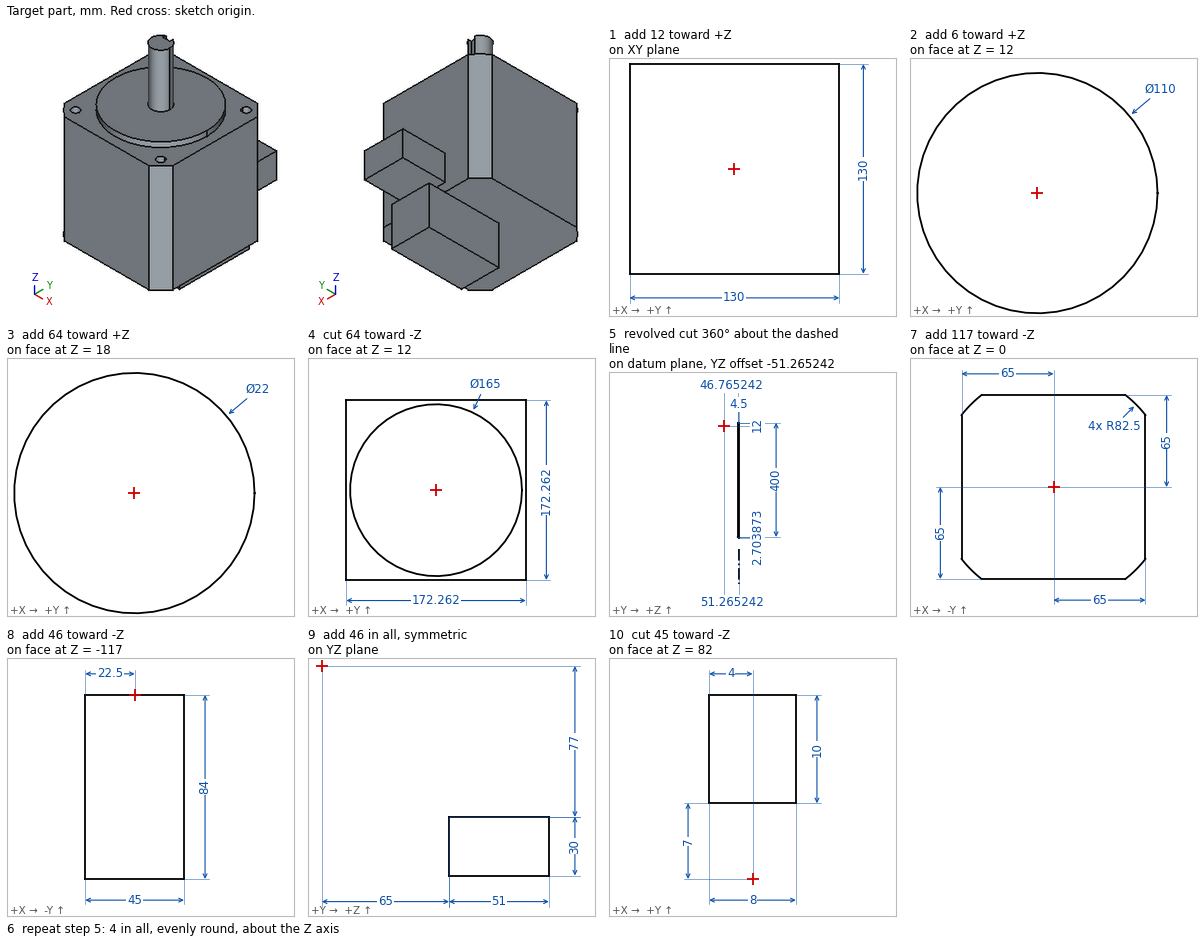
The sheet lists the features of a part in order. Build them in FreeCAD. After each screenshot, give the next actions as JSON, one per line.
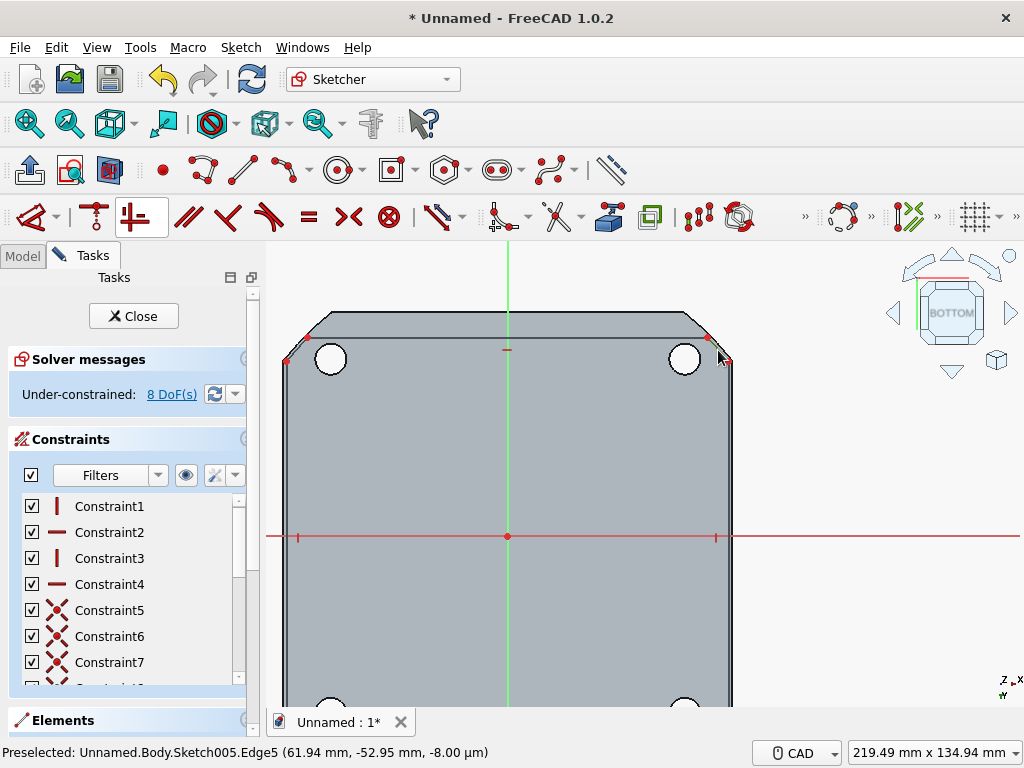
{"action": "scroll", "coordinate": [301, 345], "scroll_direction": "up", "scroll_amount": 2}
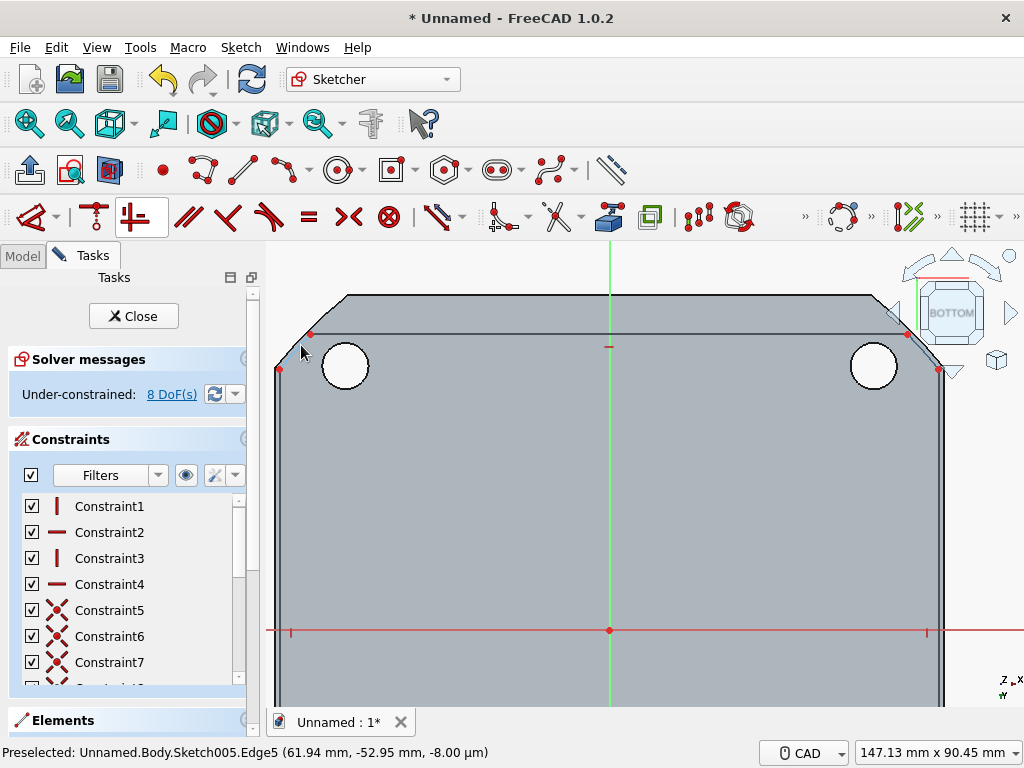
{"action": "left_click", "coordinate": [301, 345]}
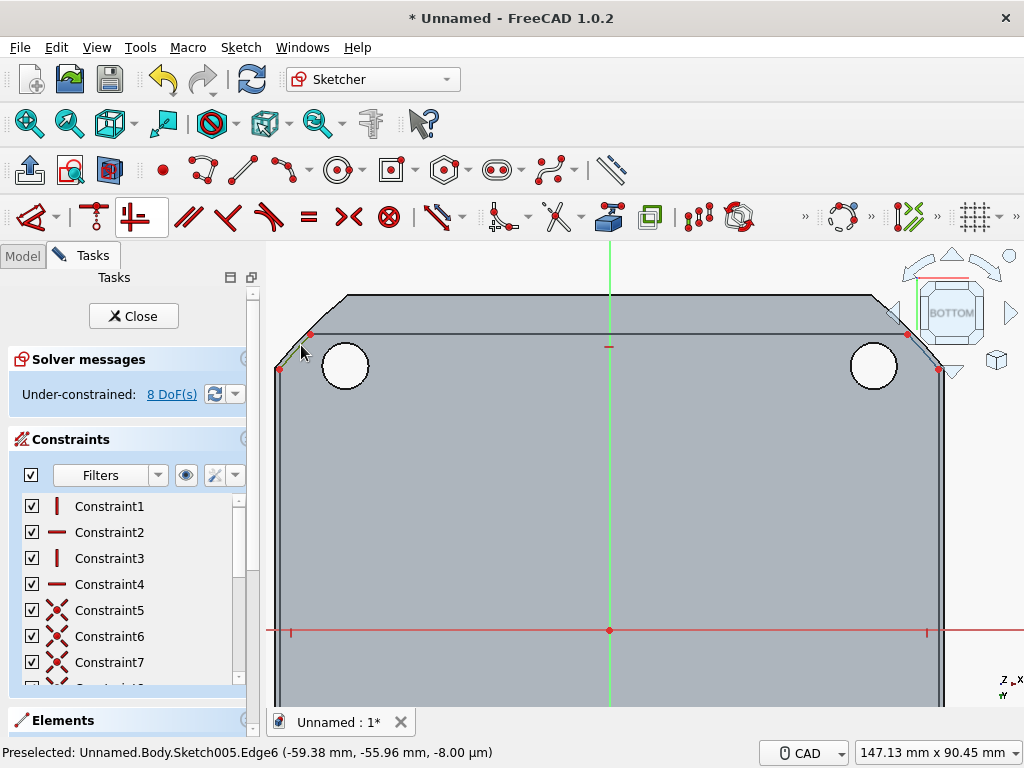
{"action": "scroll", "coordinate": [550, 347], "scroll_direction": "down", "scroll_amount": 4}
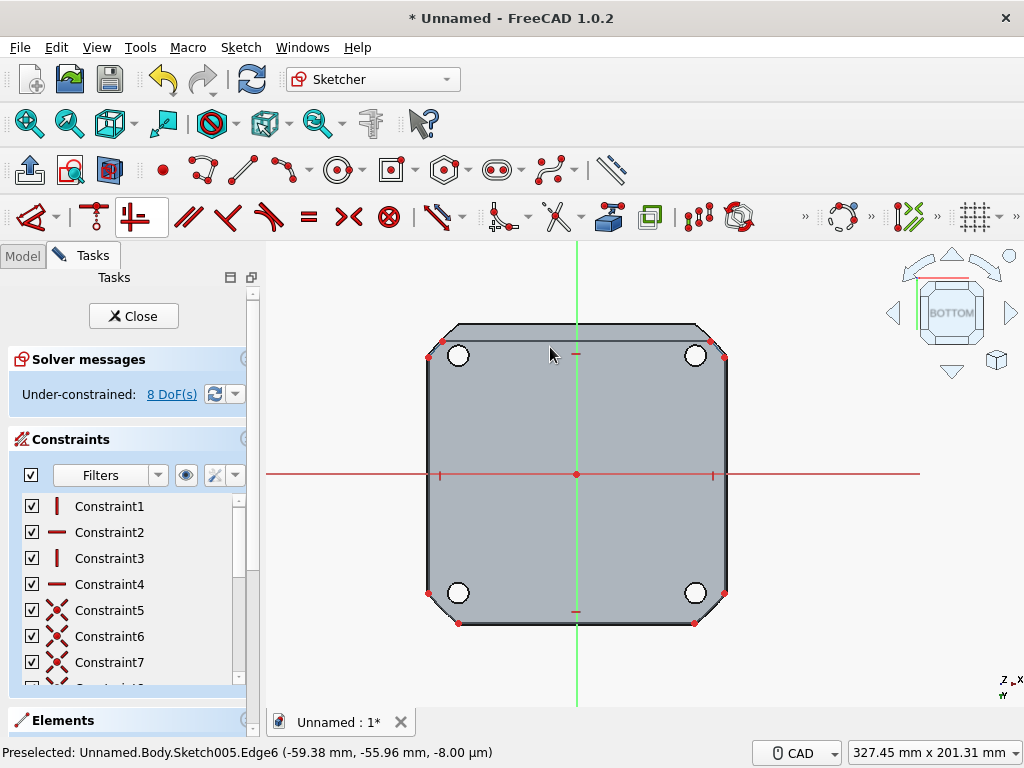
{"action": "left_click", "coordinate": [437, 603]}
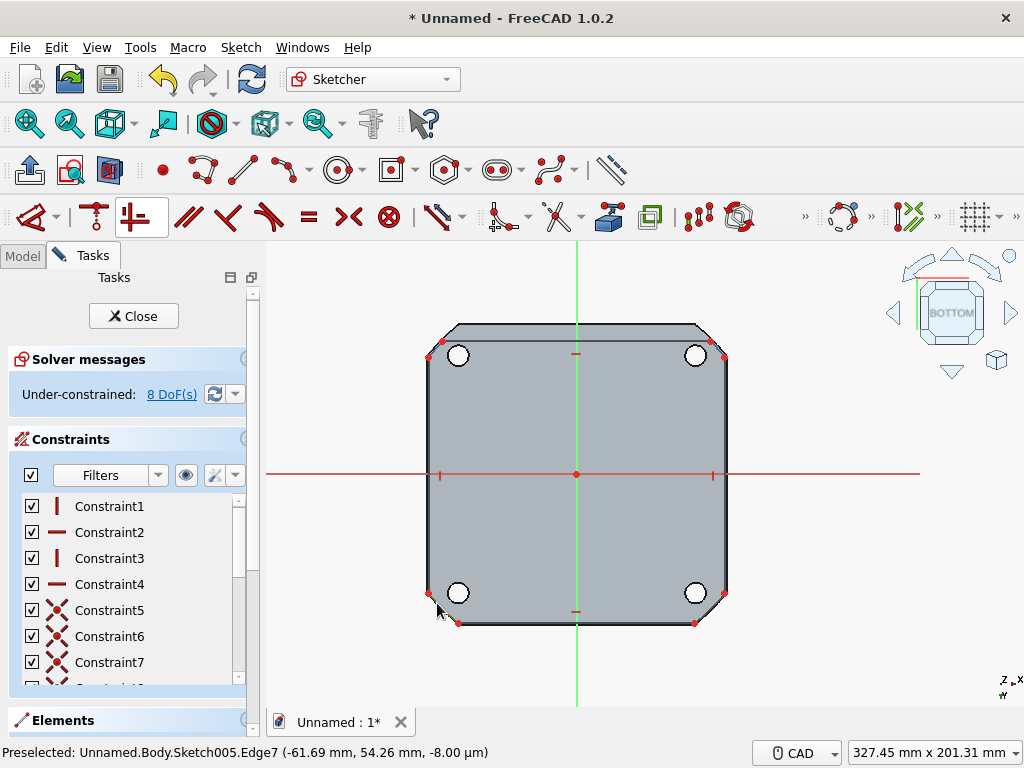
{"action": "left_click", "coordinate": [704, 615]}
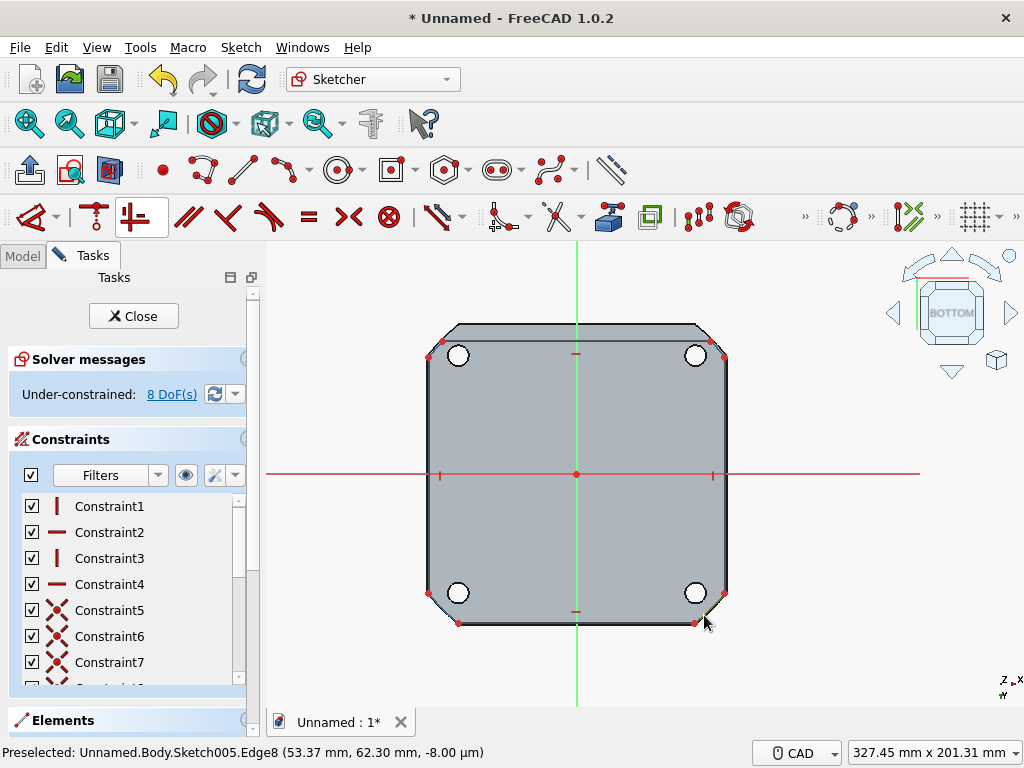
{"action": "left_click", "coordinate": [310, 218]}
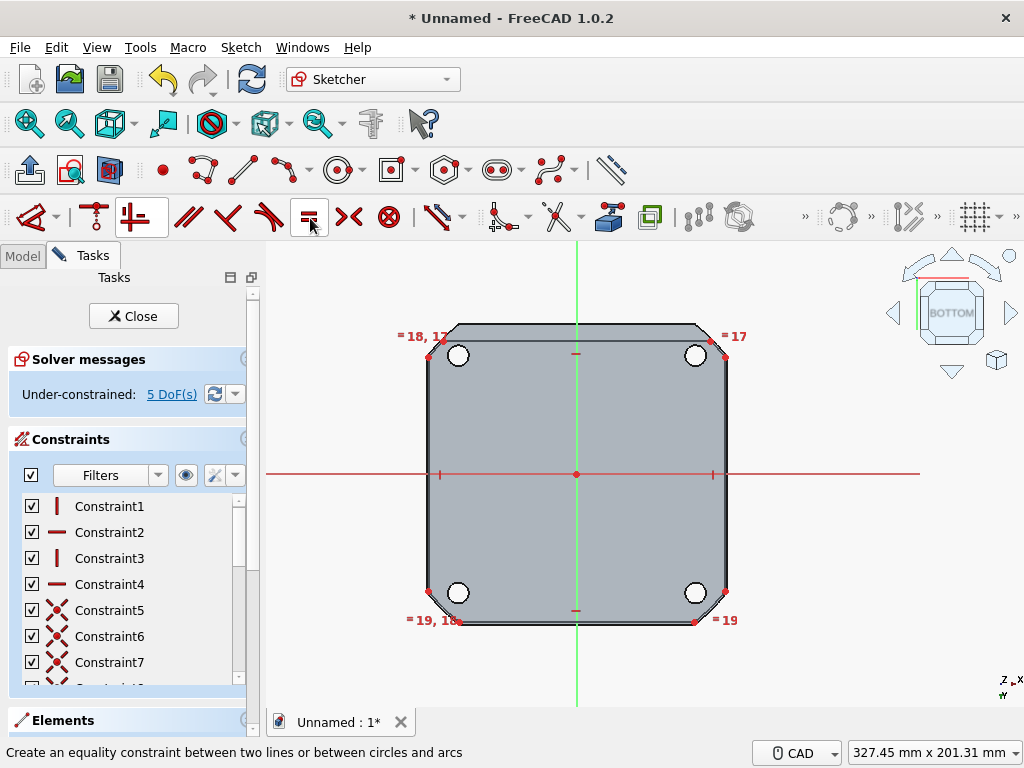
{"action": "left_click", "coordinate": [32, 218]}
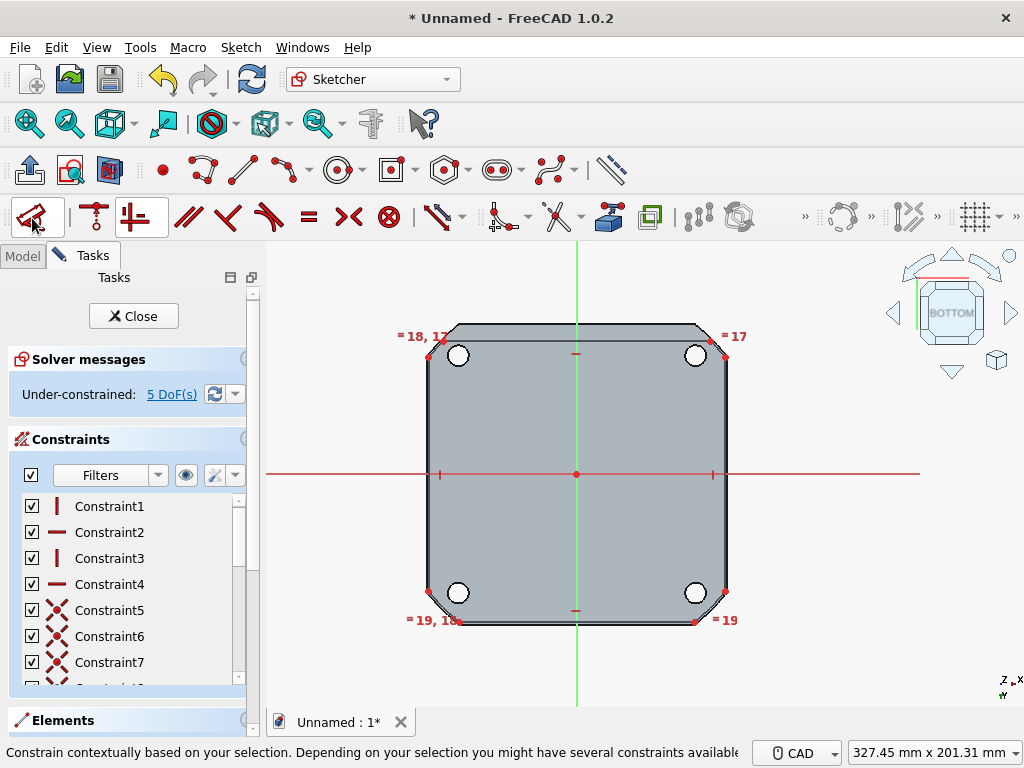
{"action": "scroll", "coordinate": [718, 349], "scroll_direction": "up", "scroll_amount": 2}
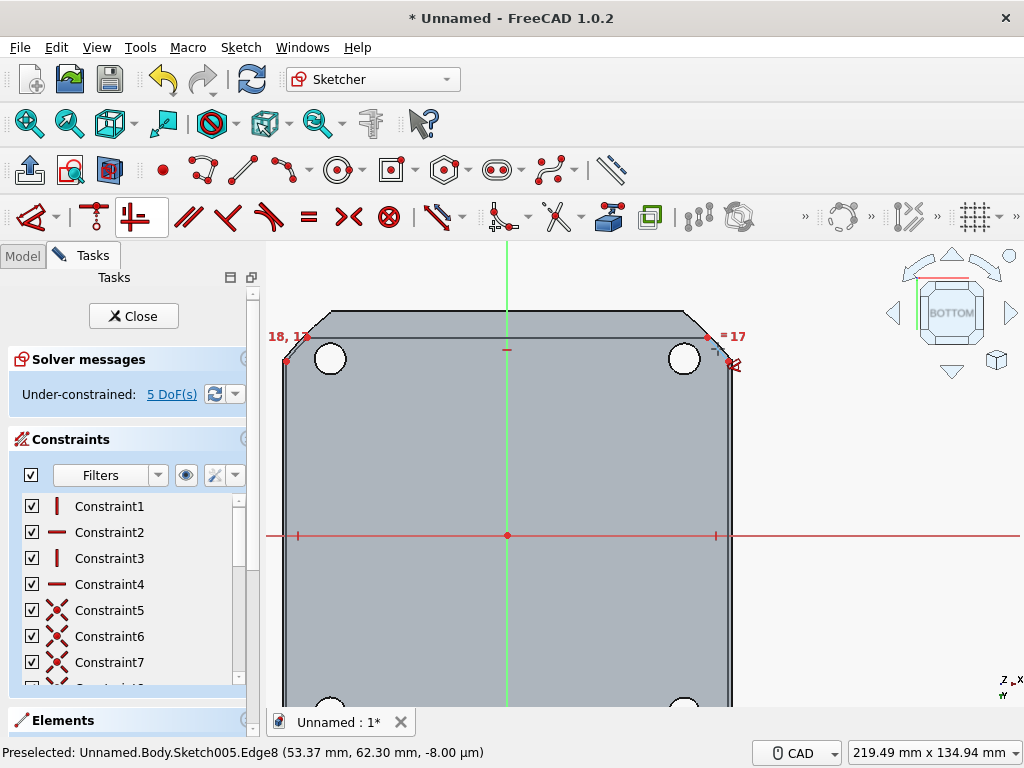
{"action": "left_click", "coordinate": [718, 349]}
{"action": "left_click", "coordinate": [742, 328]}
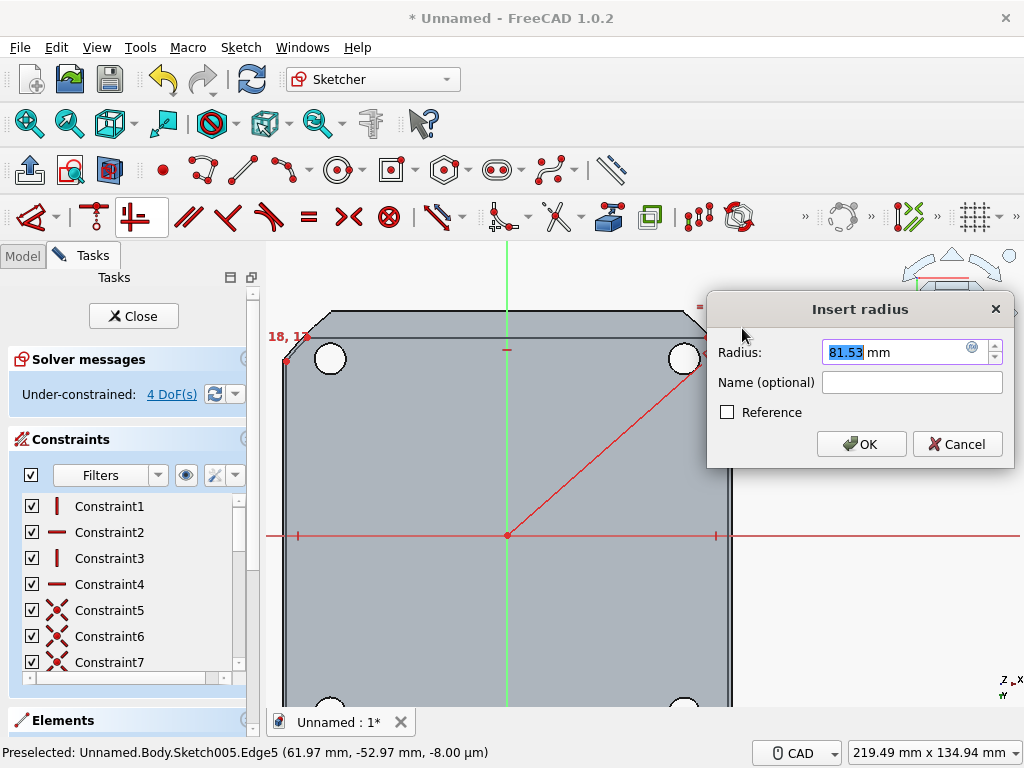
{"action": "type", "text": "82.5"}
{"action": "key", "text": "Return"}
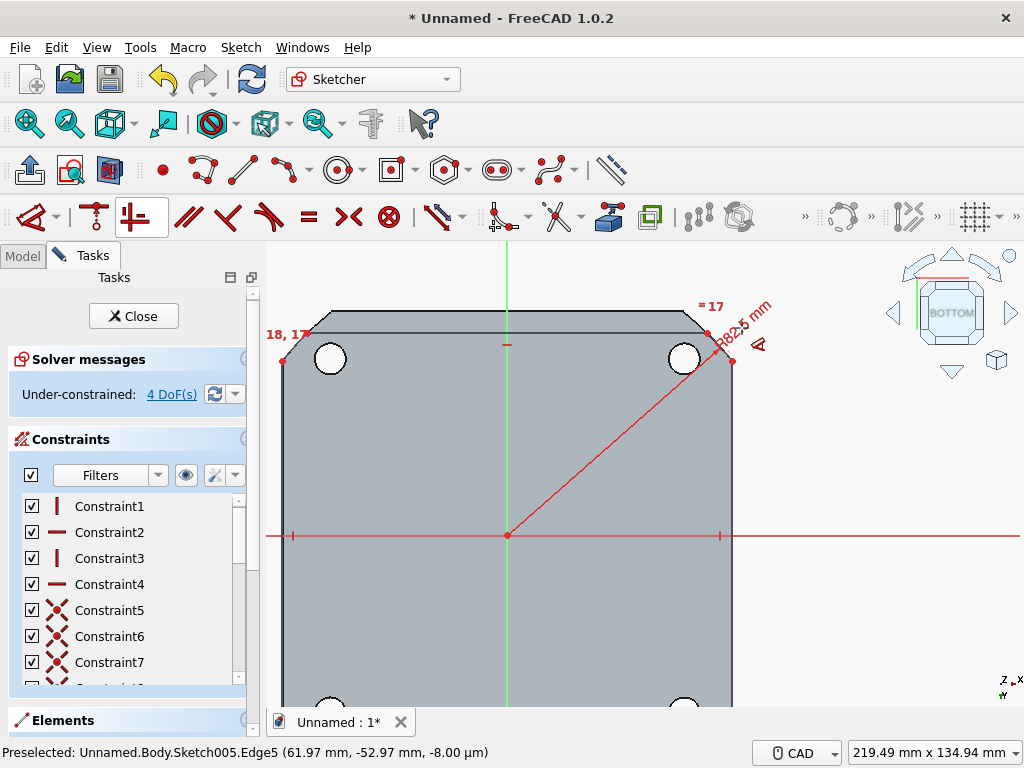
{"action": "scroll", "coordinate": [717, 348], "scroll_direction": "down", "scroll_amount": 2}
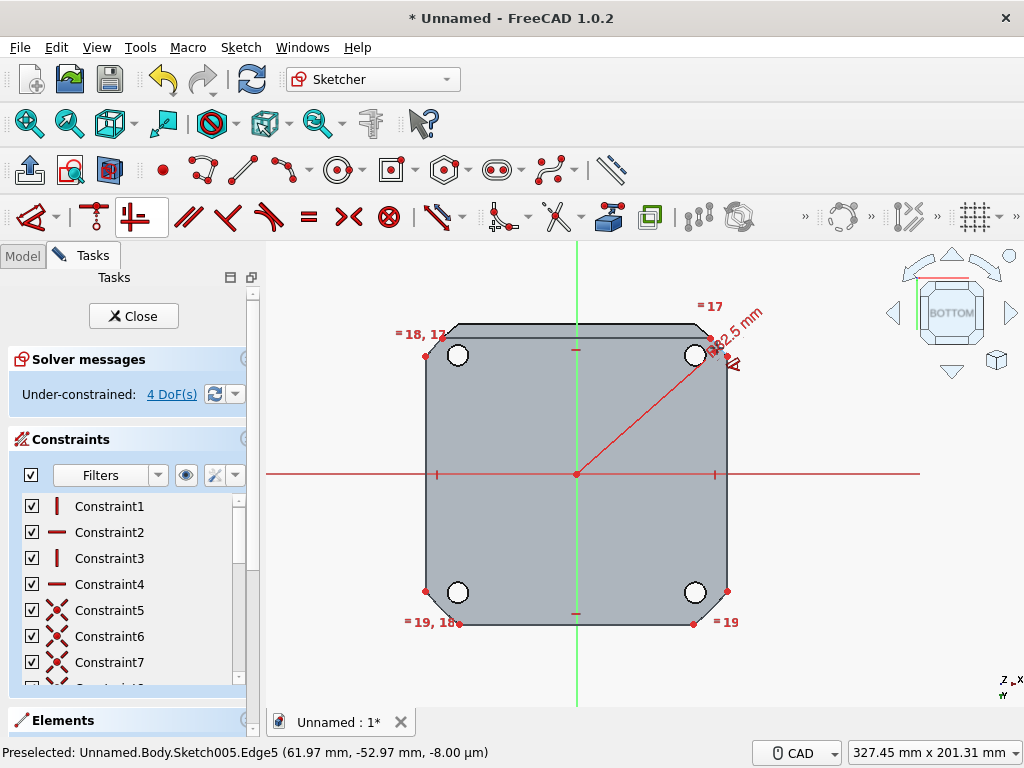
{"action": "left_click", "coordinate": [727, 591]}
{"action": "left_click", "coordinate": [652, 440]}